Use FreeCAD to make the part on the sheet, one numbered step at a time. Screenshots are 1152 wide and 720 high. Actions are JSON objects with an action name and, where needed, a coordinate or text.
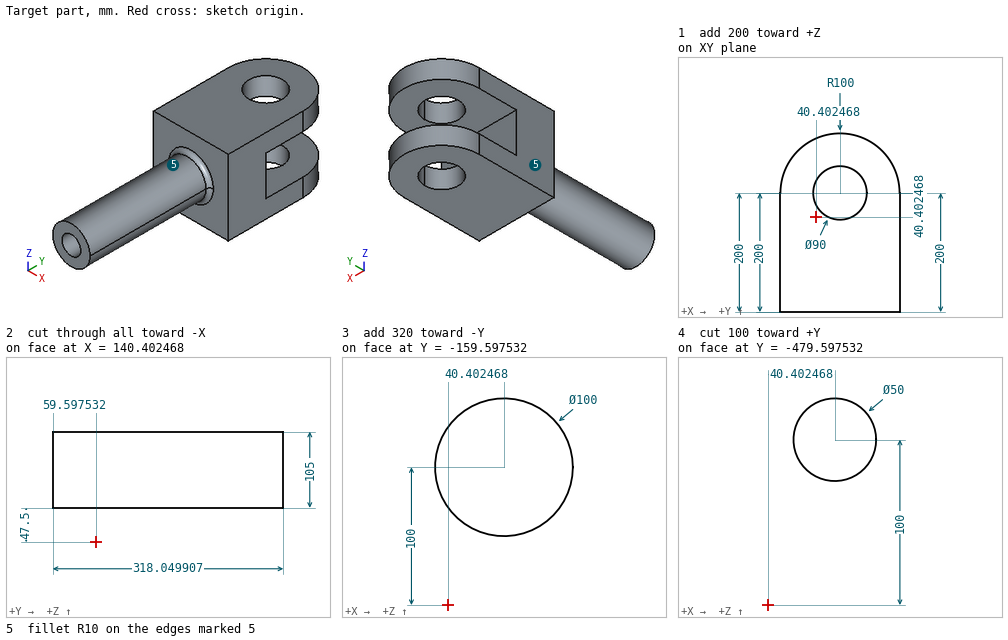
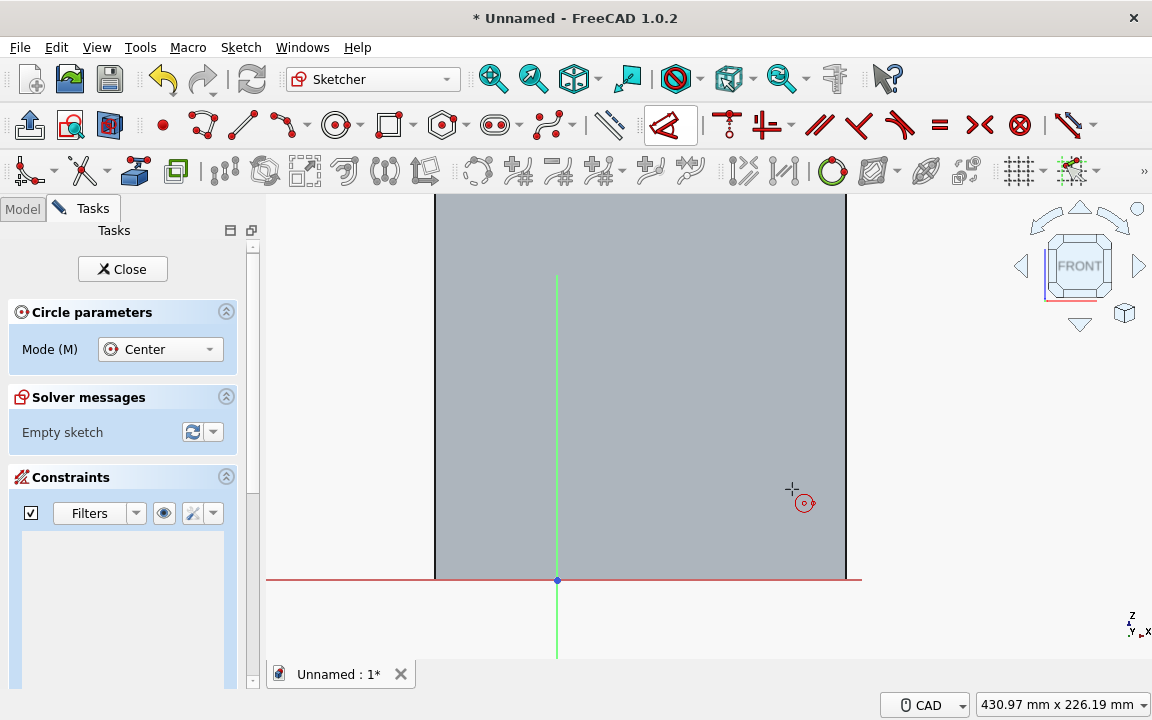
{"action": "left_click", "coordinate": [640, 375]}
{"action": "mouse_move", "coordinate": [713, 302]}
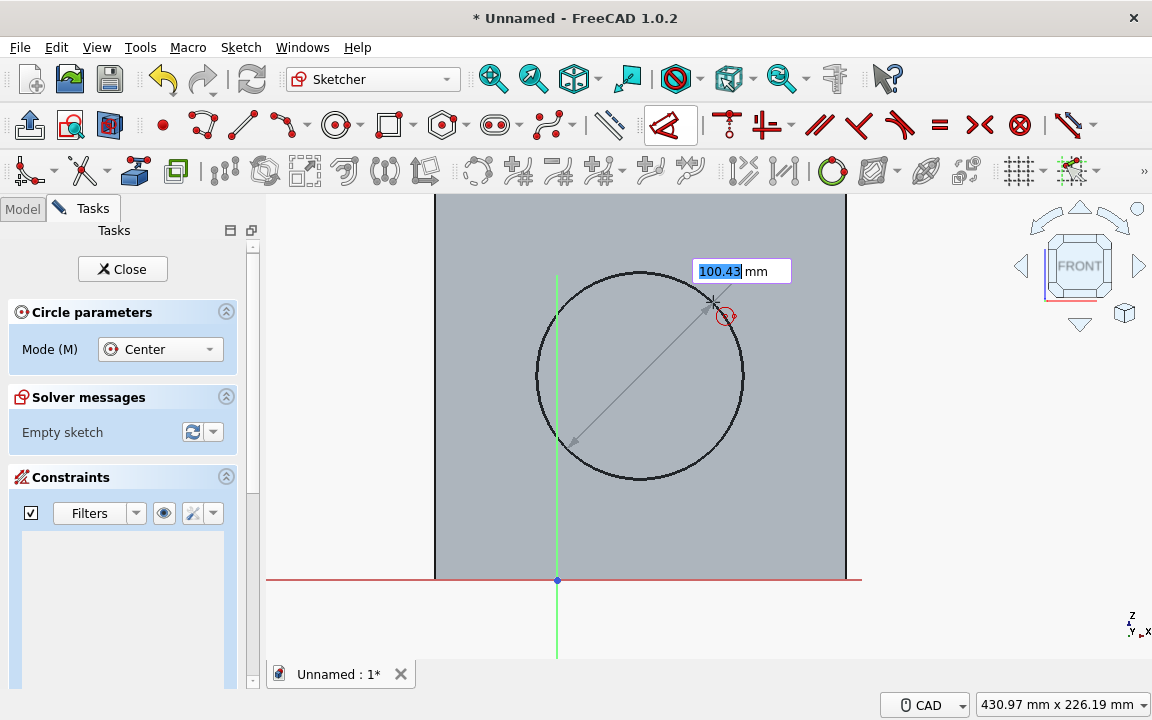
{"action": "type", "text": "100"}
{"action": "key", "text": "Return"}
{"action": "key", "text": "Escape"}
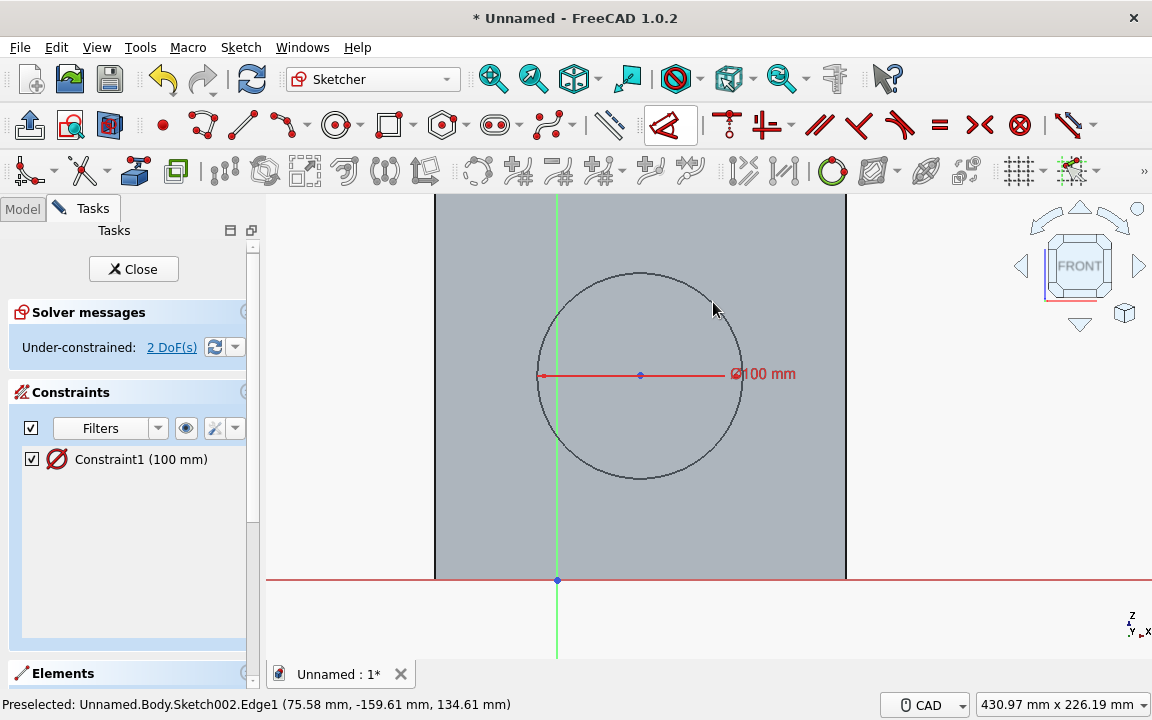
{"action": "left_click", "coordinate": [640, 376]}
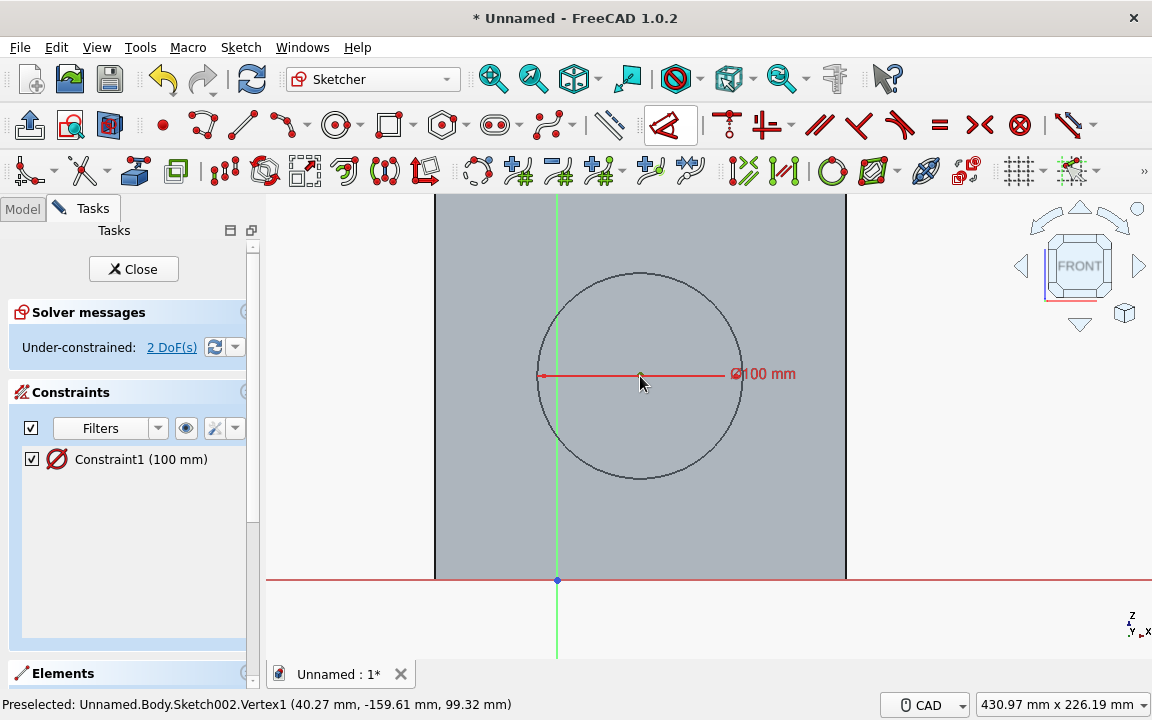
{"action": "left_click", "coordinate": [692, 126]}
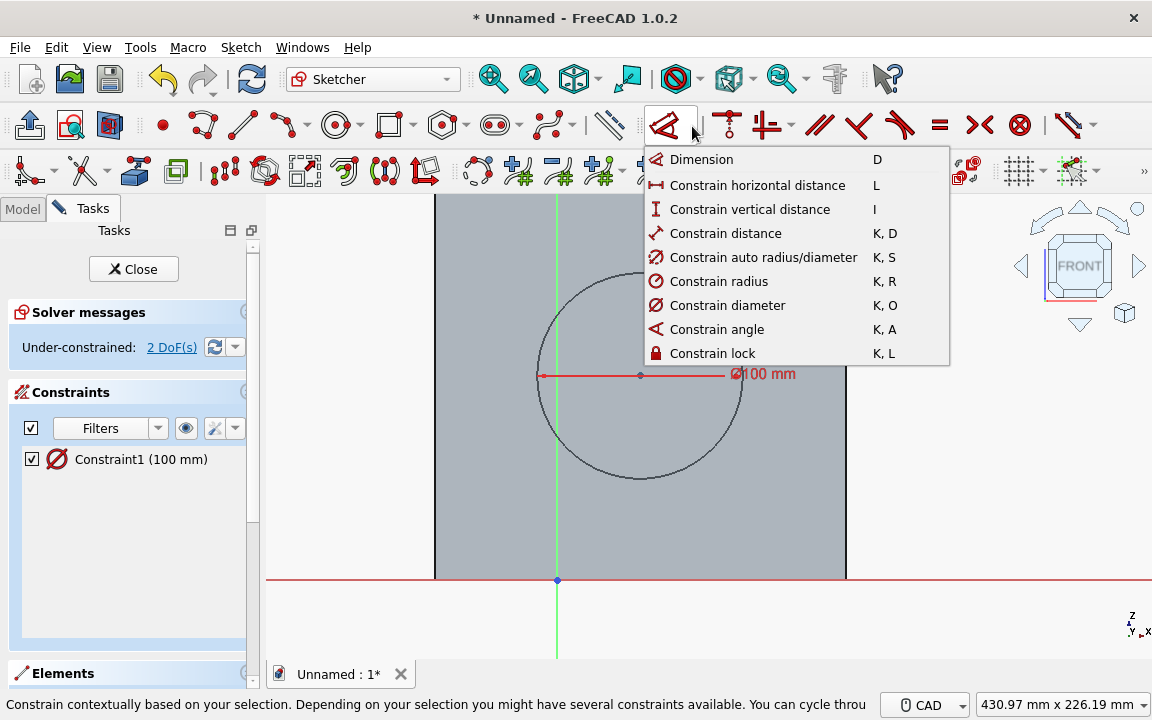
{"action": "left_click", "coordinate": [797, 209]}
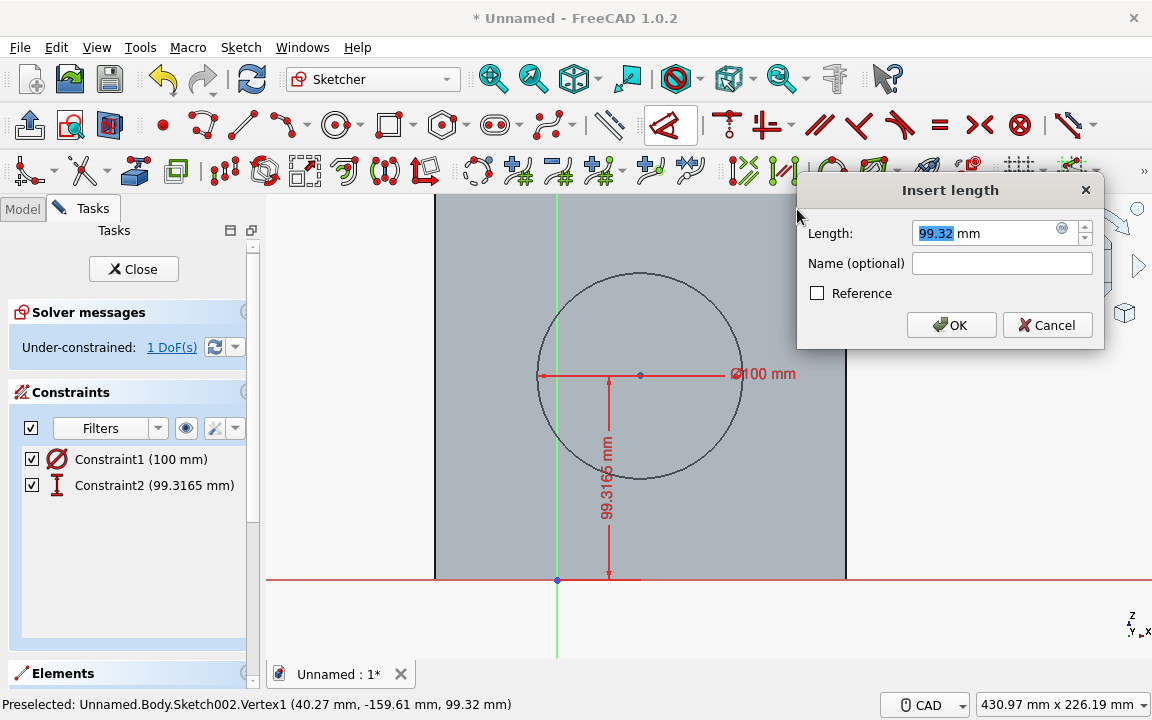
{"action": "type", "text": "100"}
{"action": "key", "text": "Return"}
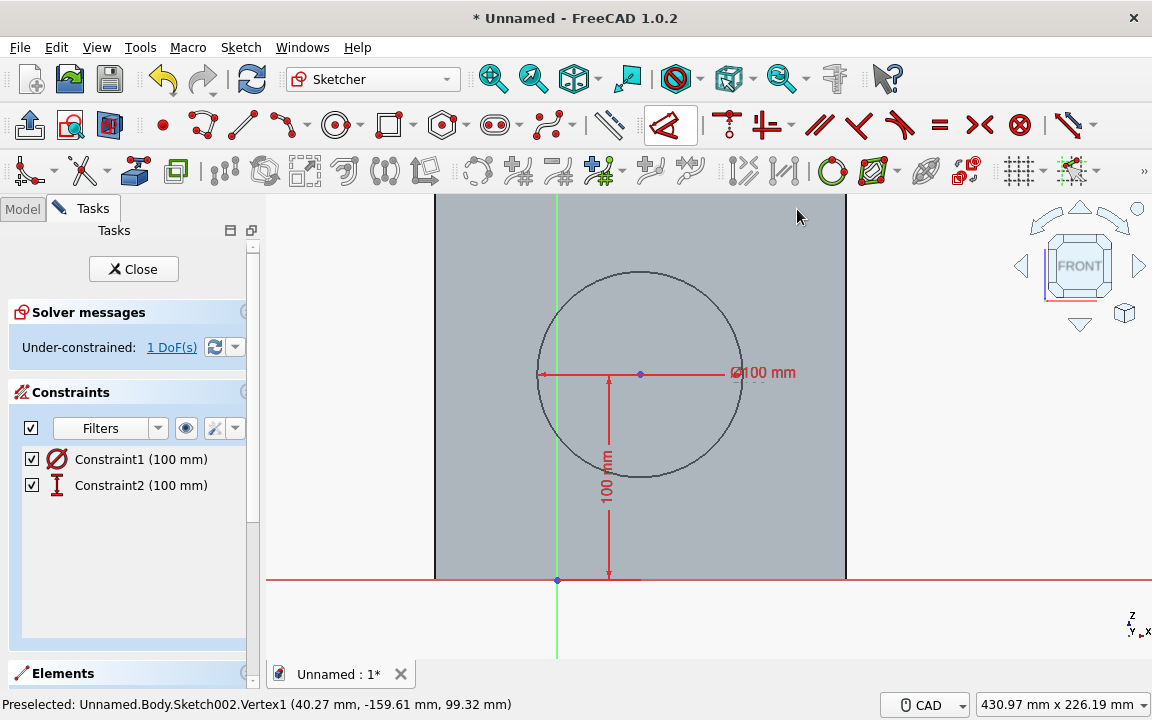
{"action": "left_click", "coordinate": [640, 375]}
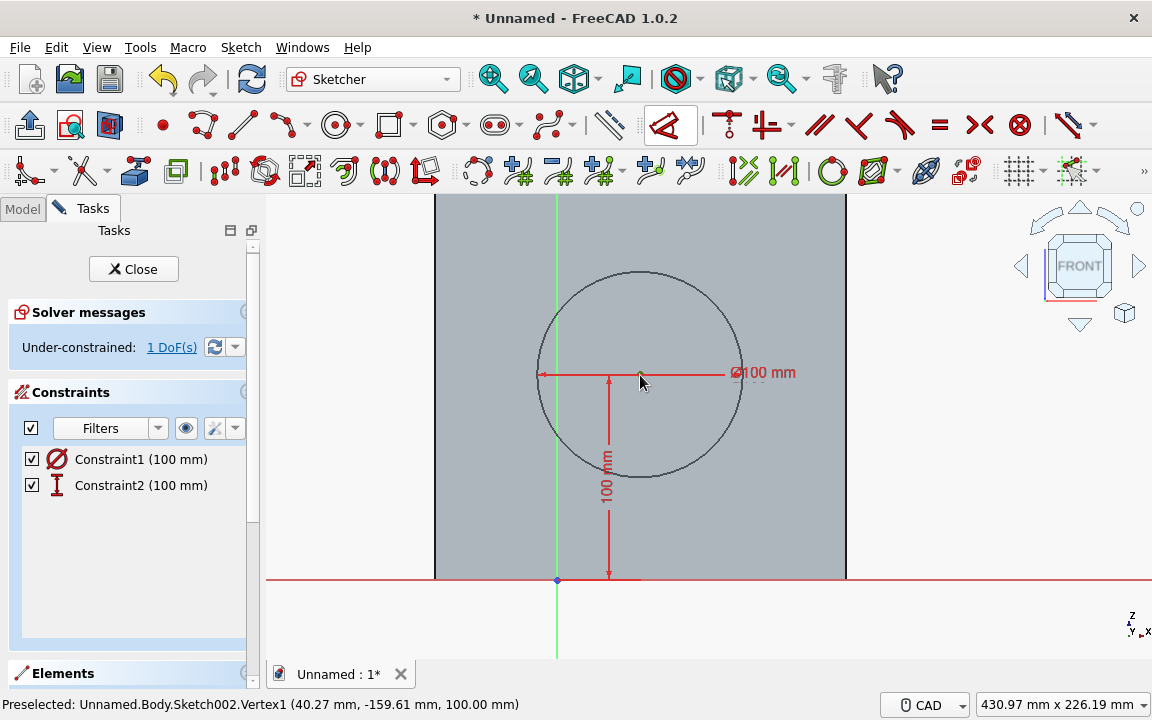
{"action": "left_click", "coordinate": [692, 126]}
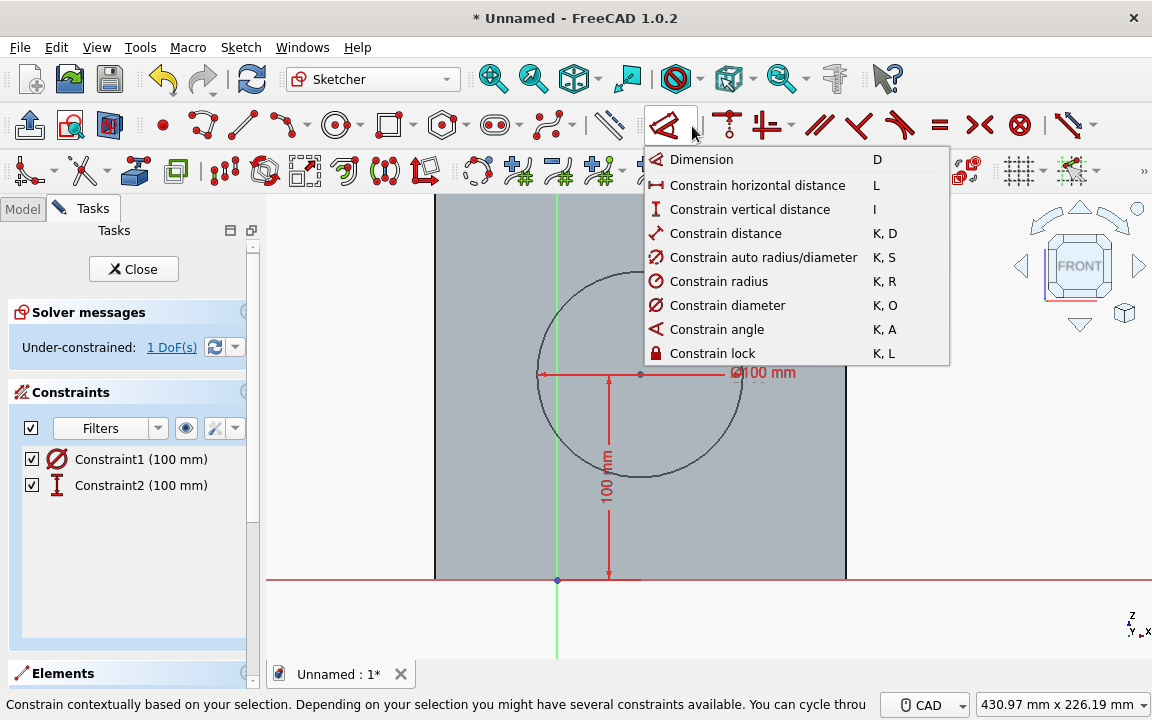
{"action": "left_click", "coordinate": [797, 185]}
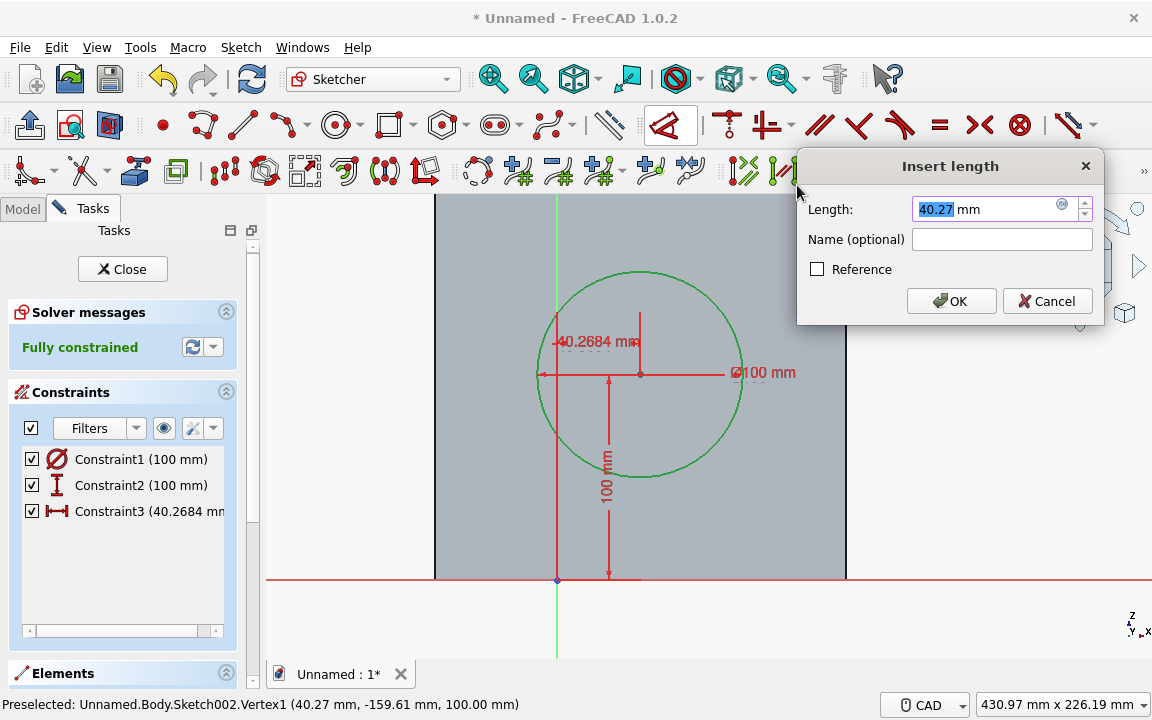
{"action": "type", "text": "40.402468"}
{"action": "key", "text": "Return"}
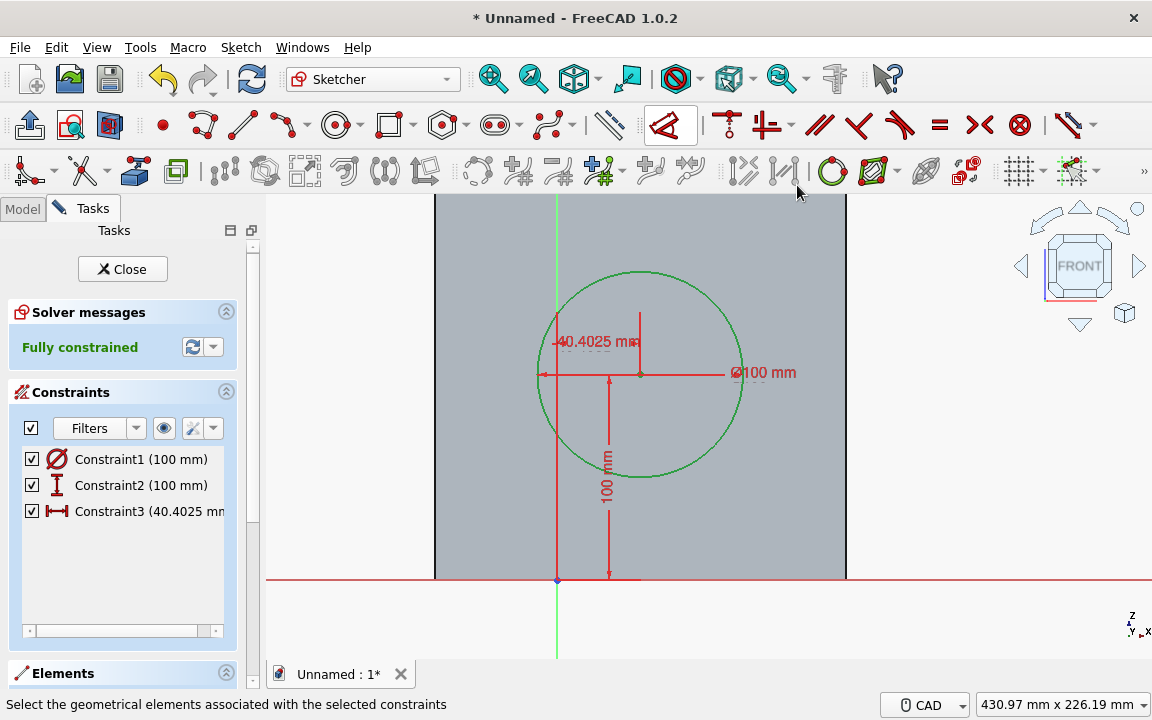
{"action": "left_click", "coordinate": [123, 269]}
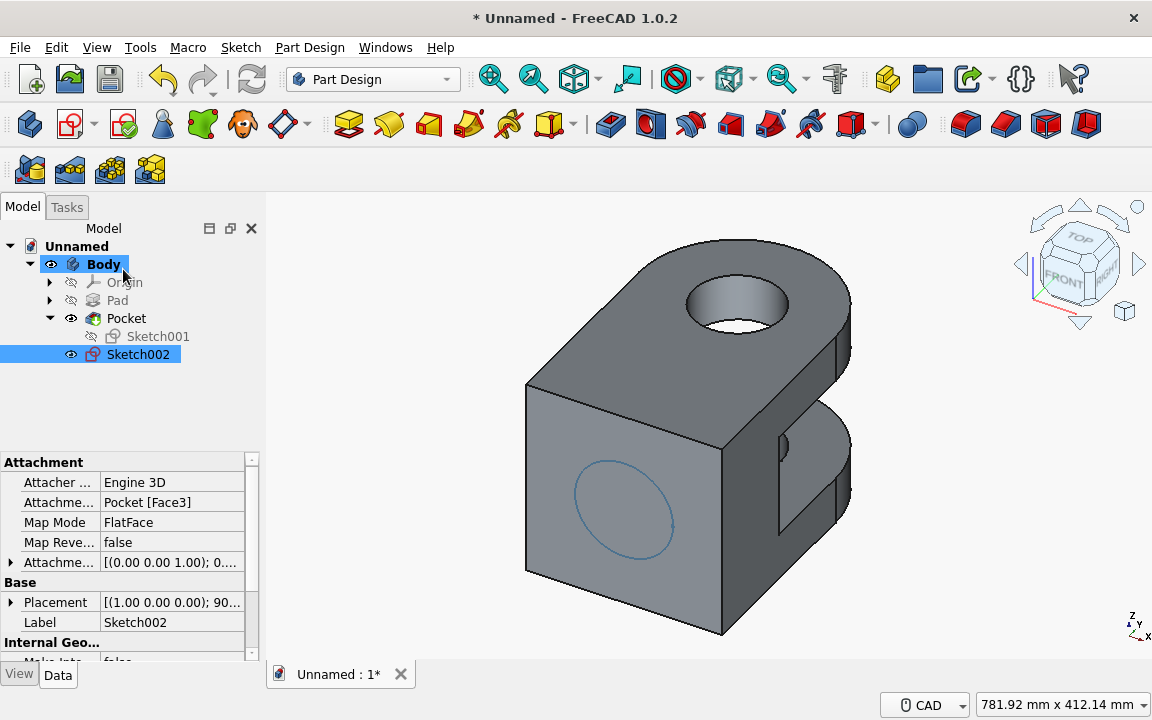
{"action": "left_click", "coordinate": [350, 124]}